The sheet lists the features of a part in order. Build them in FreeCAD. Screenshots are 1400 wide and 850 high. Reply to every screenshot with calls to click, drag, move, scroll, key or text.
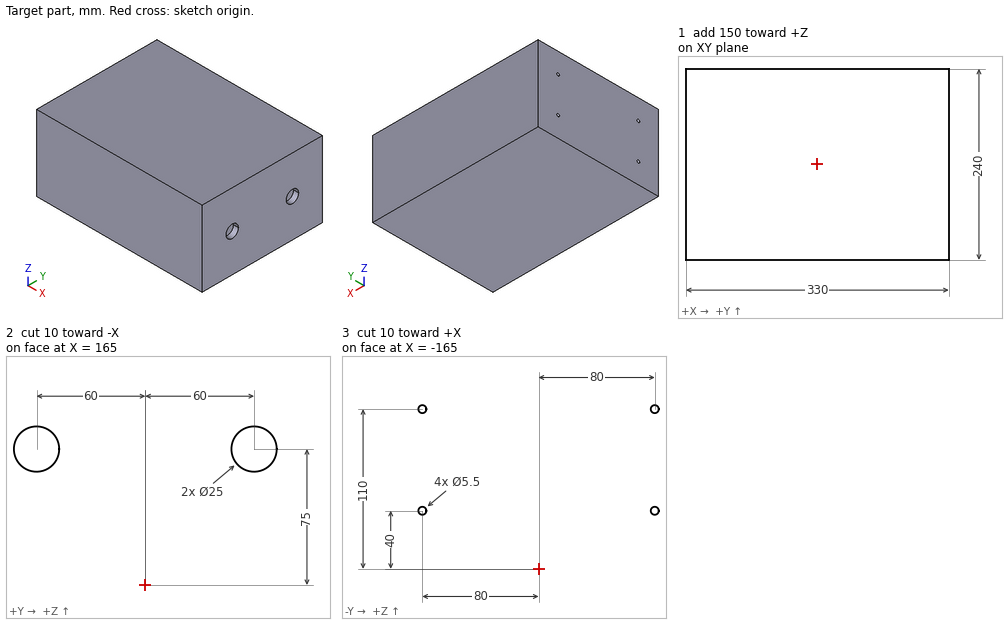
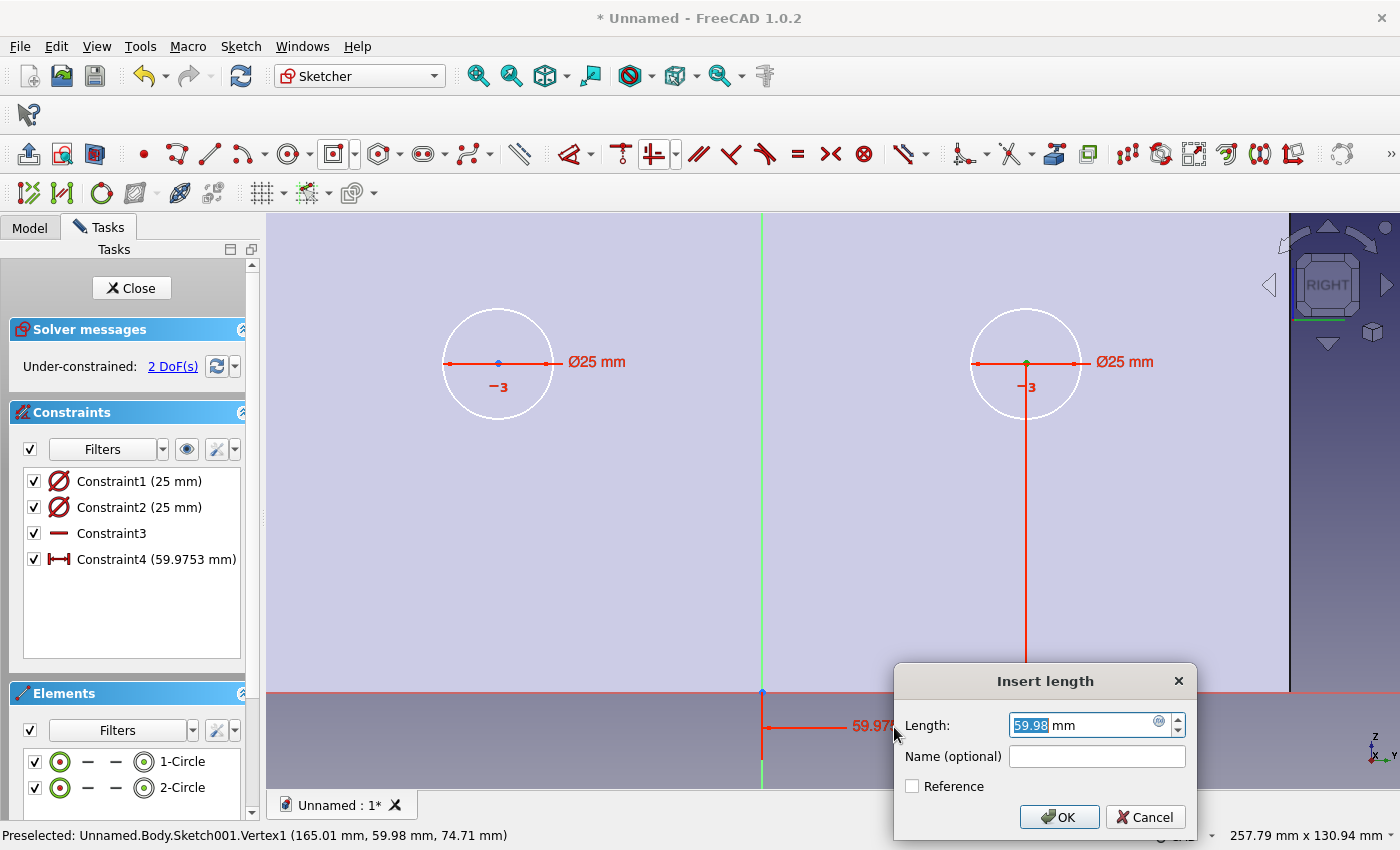
text(60)
key(Return)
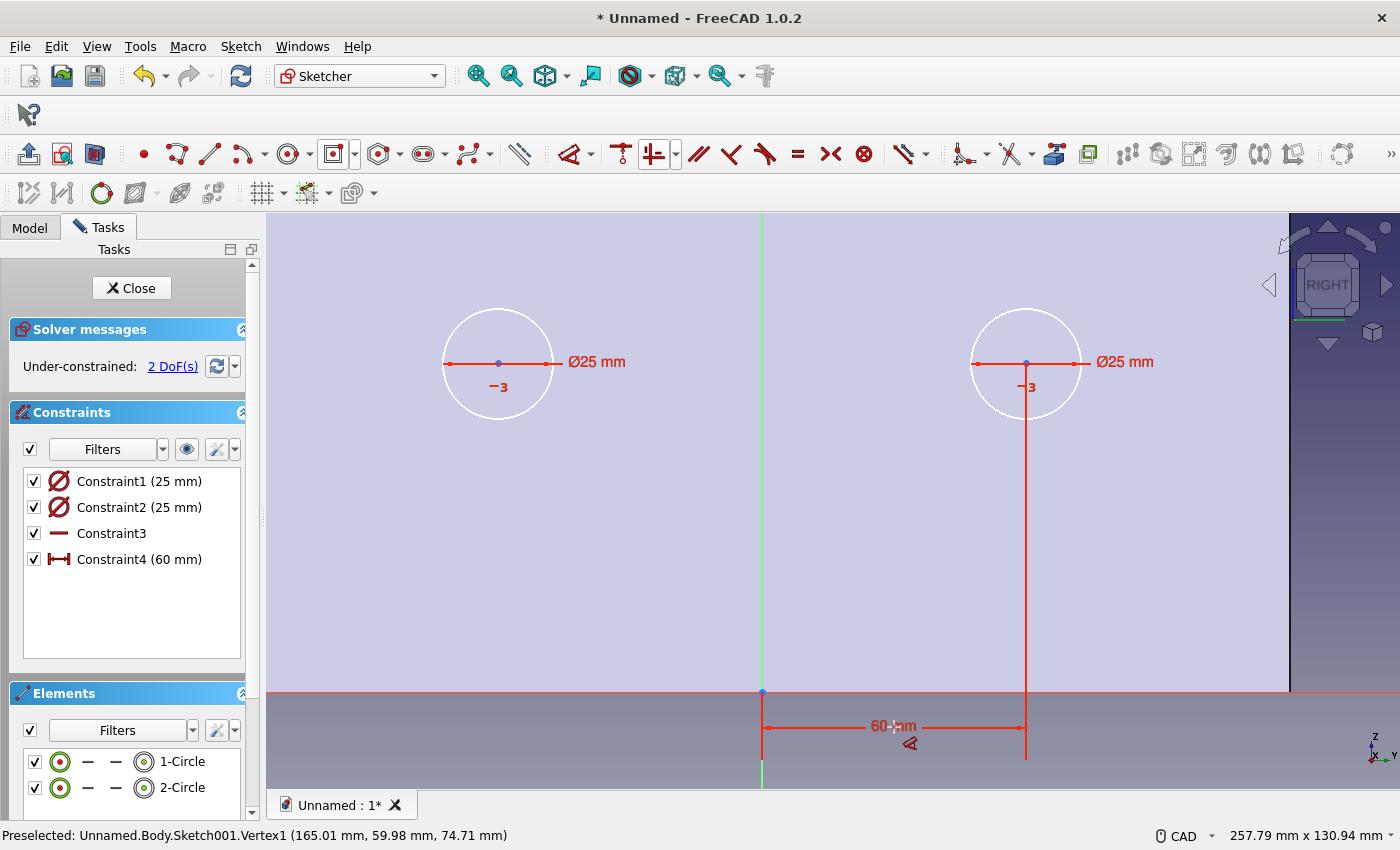
click(1026, 364)
click(1060, 528)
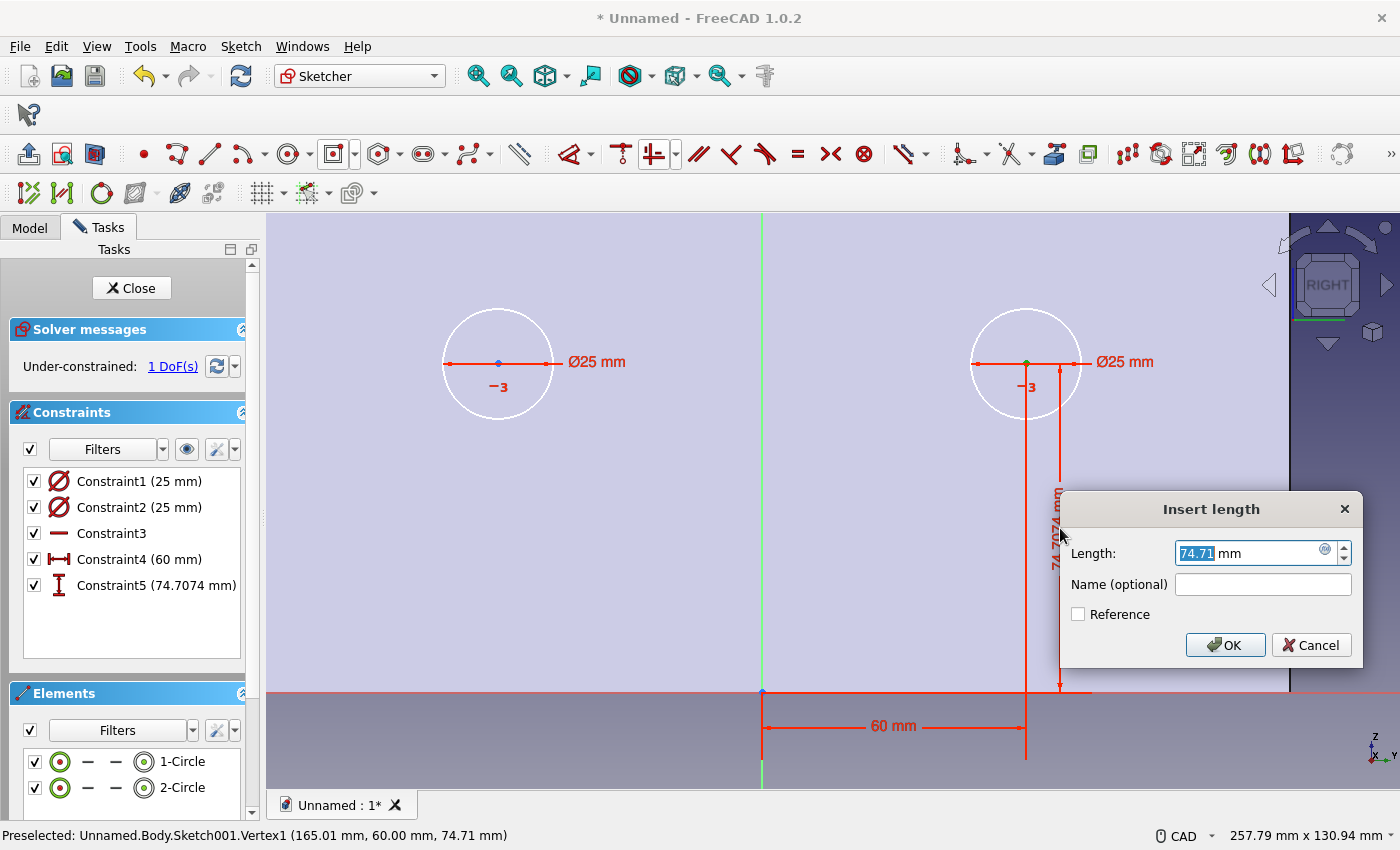
text(75)
key(Return)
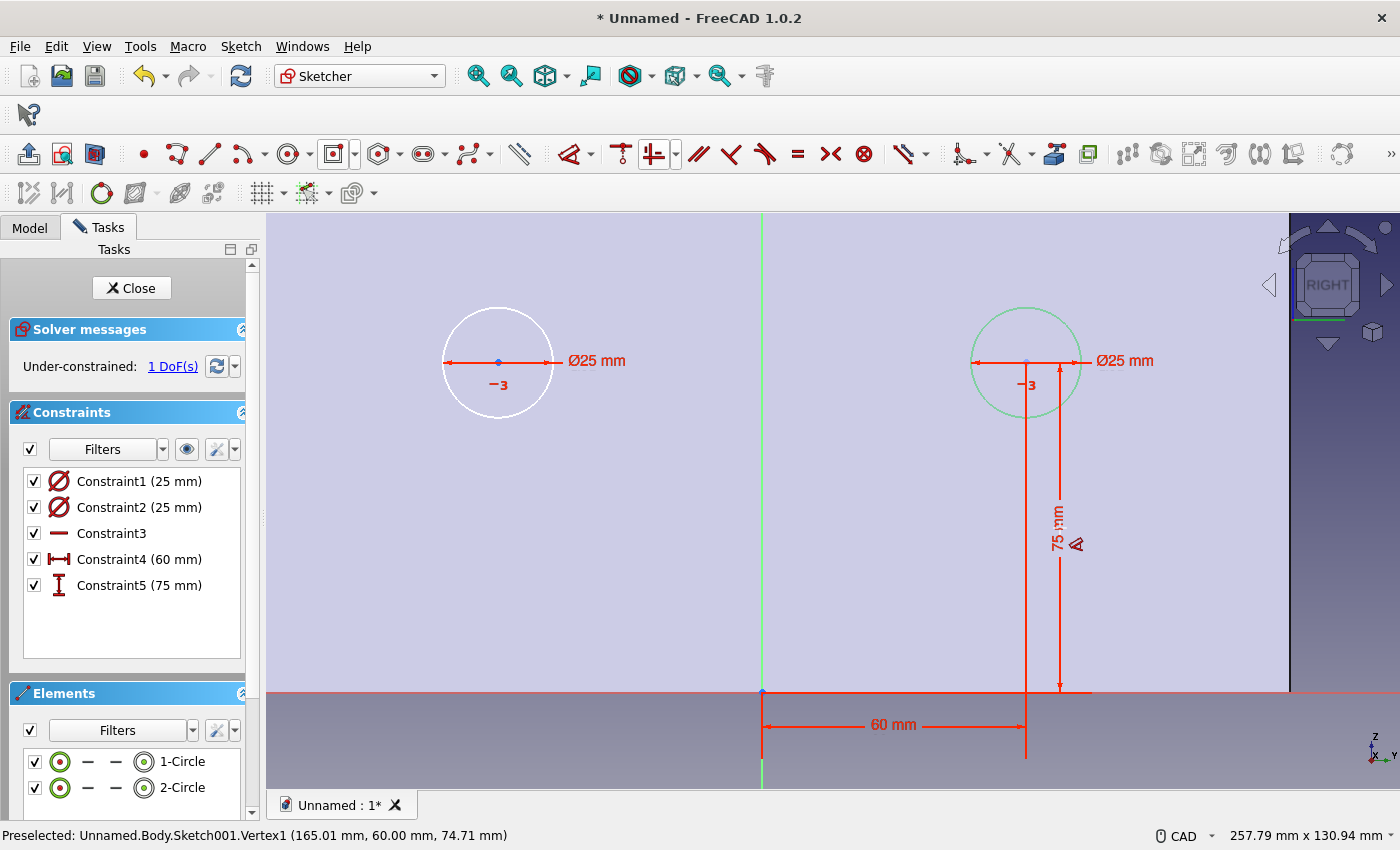
click(498, 363)
click(630, 727)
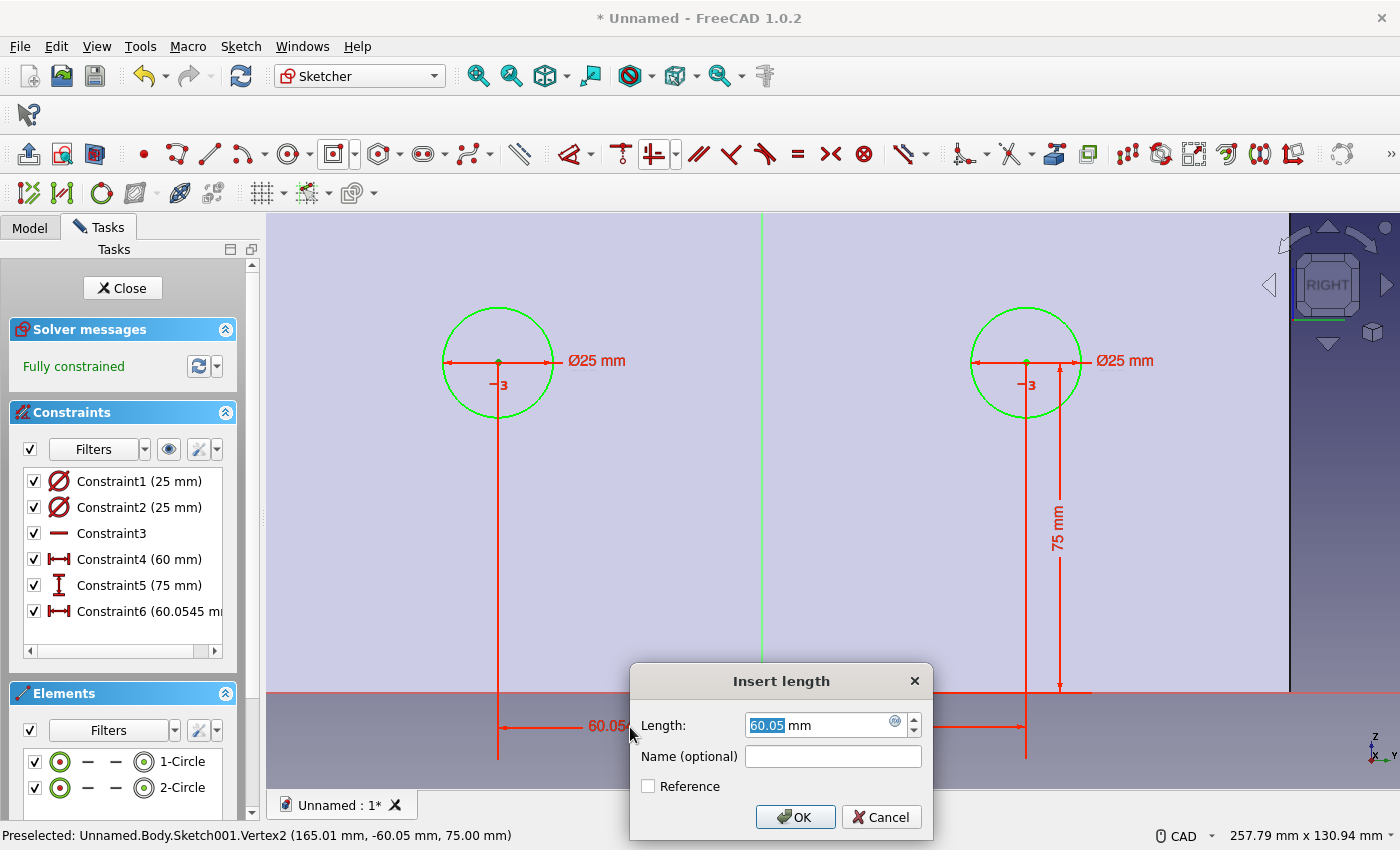
text(60)
key(Return)
key(Escape)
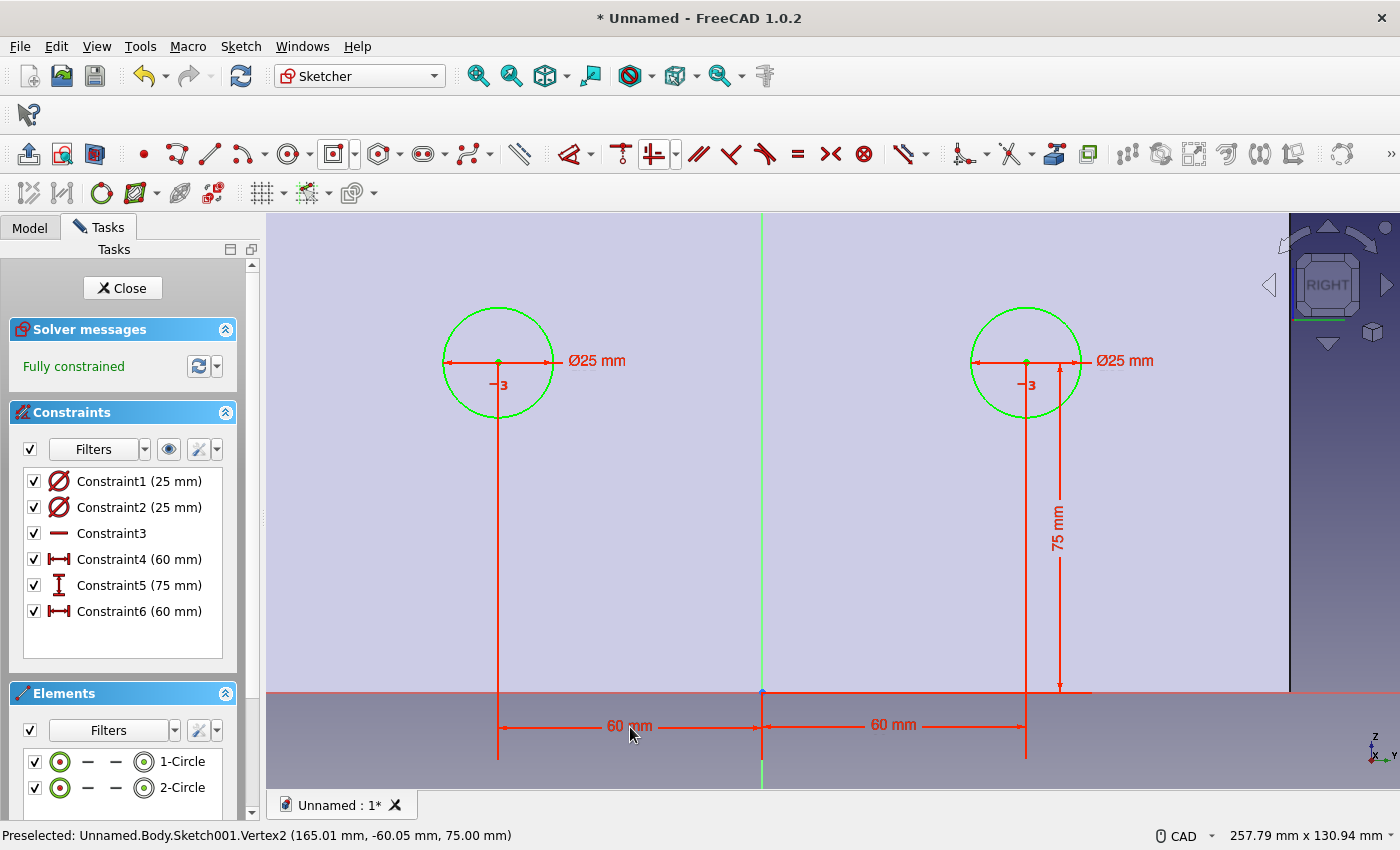
click(123, 288)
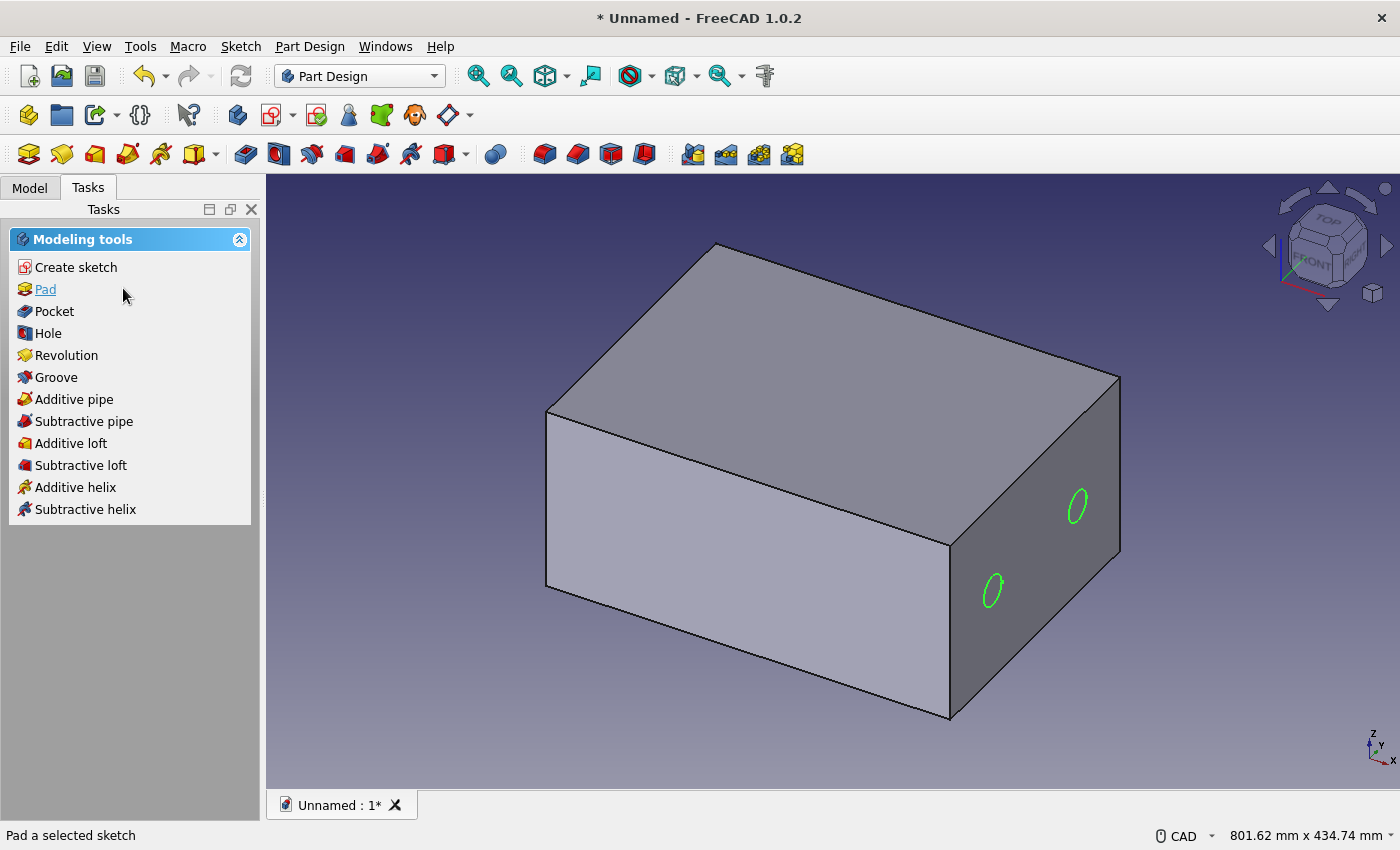
click(246, 154)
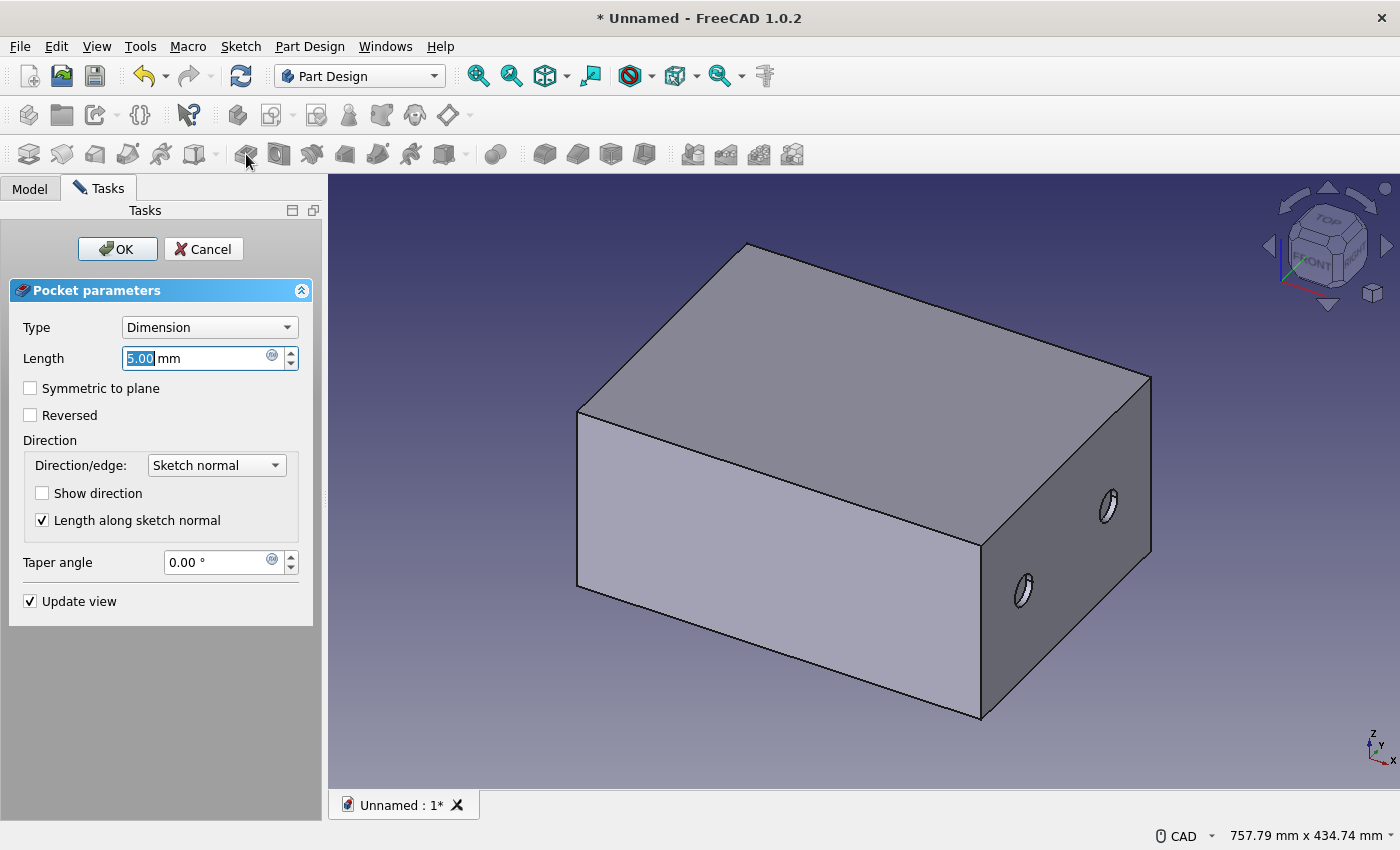
text(10)
key(Tab)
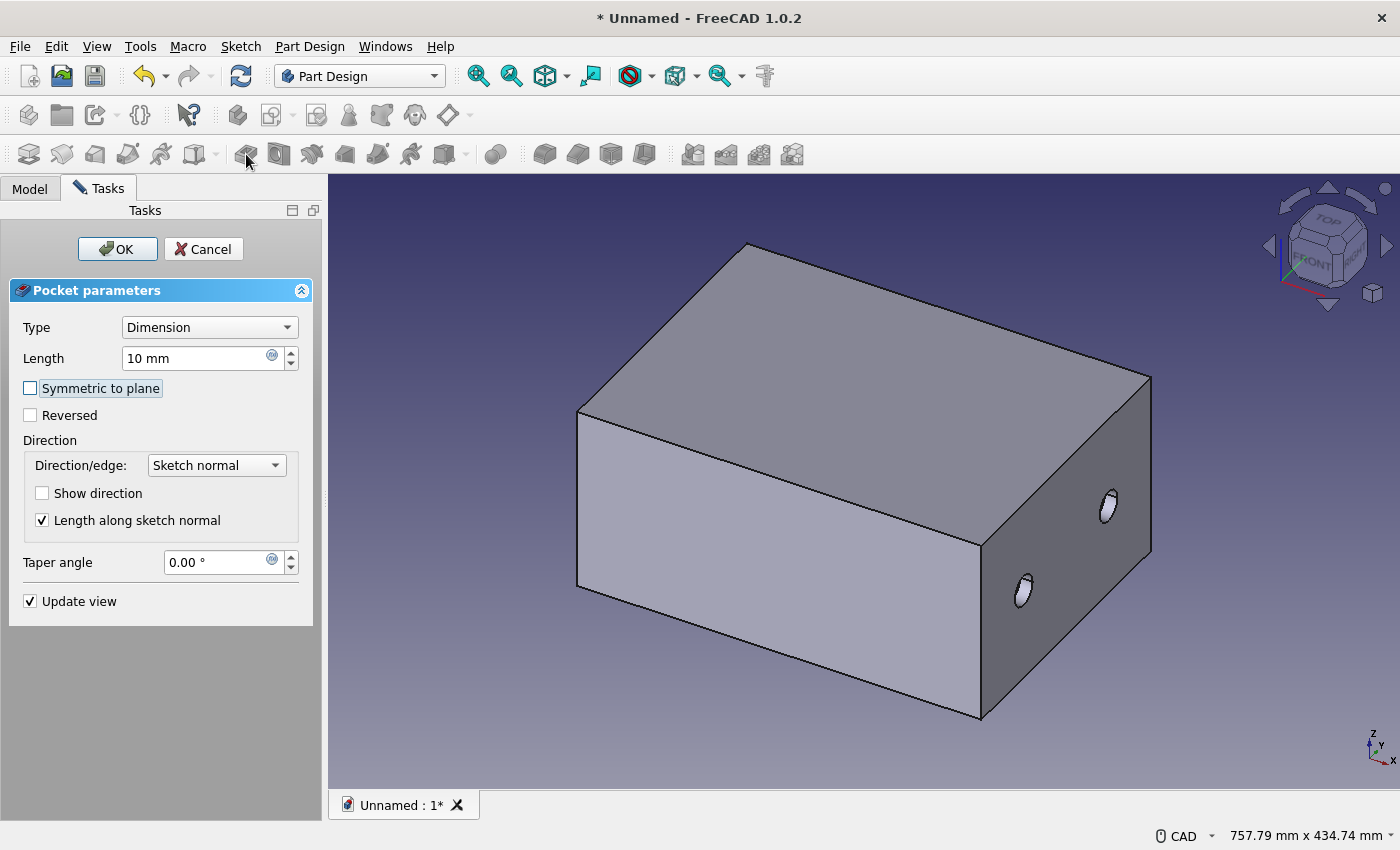
click(118, 249)